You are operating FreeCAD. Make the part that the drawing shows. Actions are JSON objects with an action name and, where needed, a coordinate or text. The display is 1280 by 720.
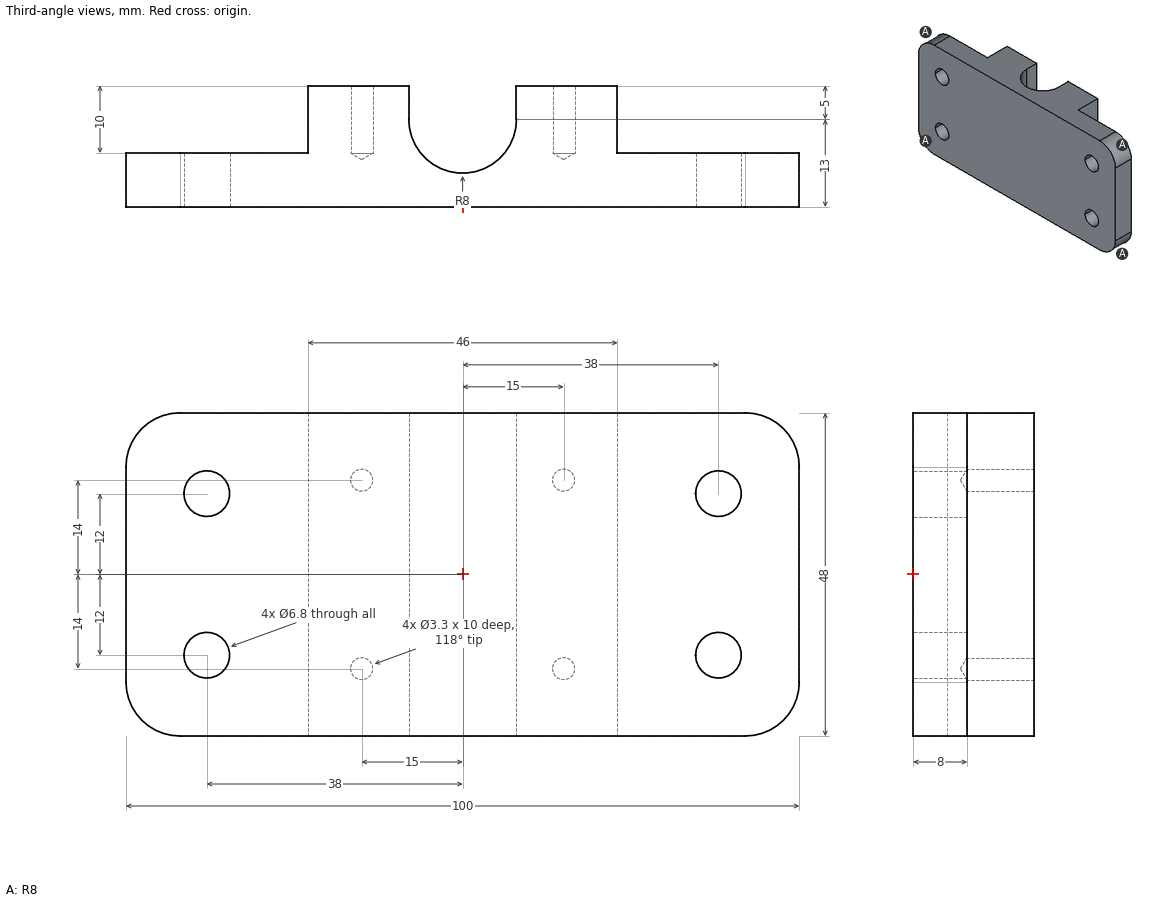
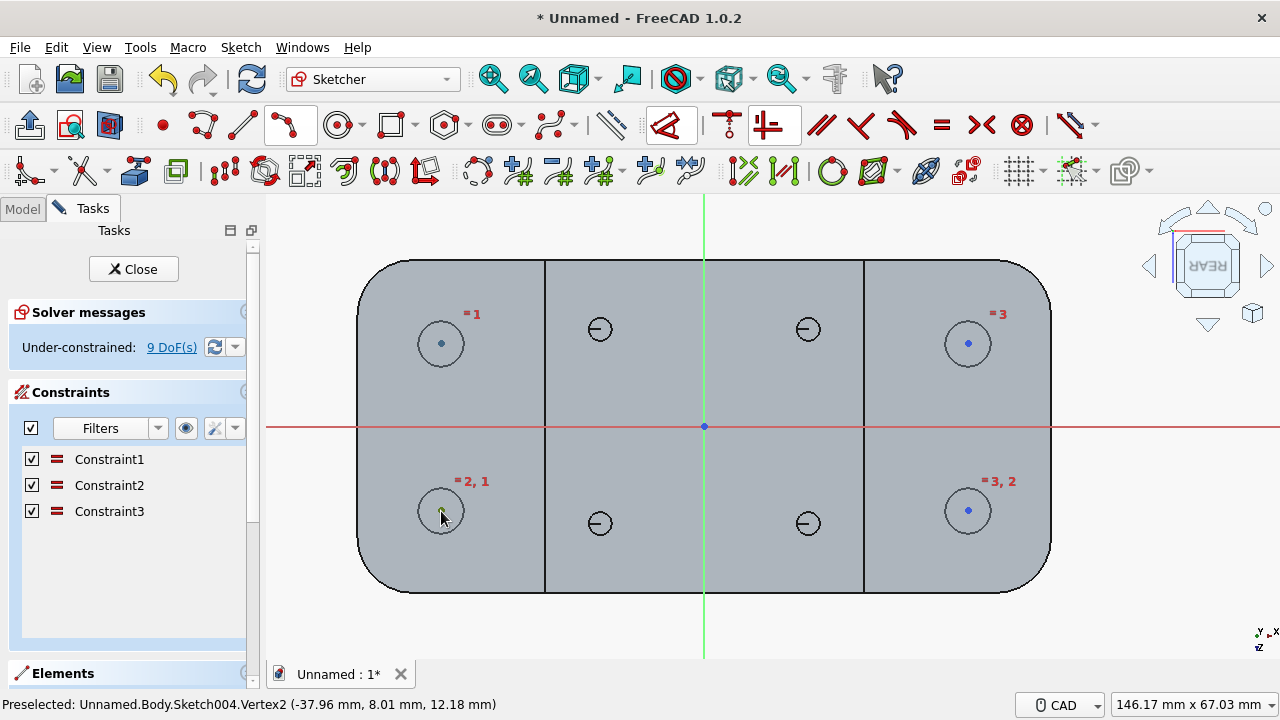
{"action": "left_click", "coordinate": [796, 126]}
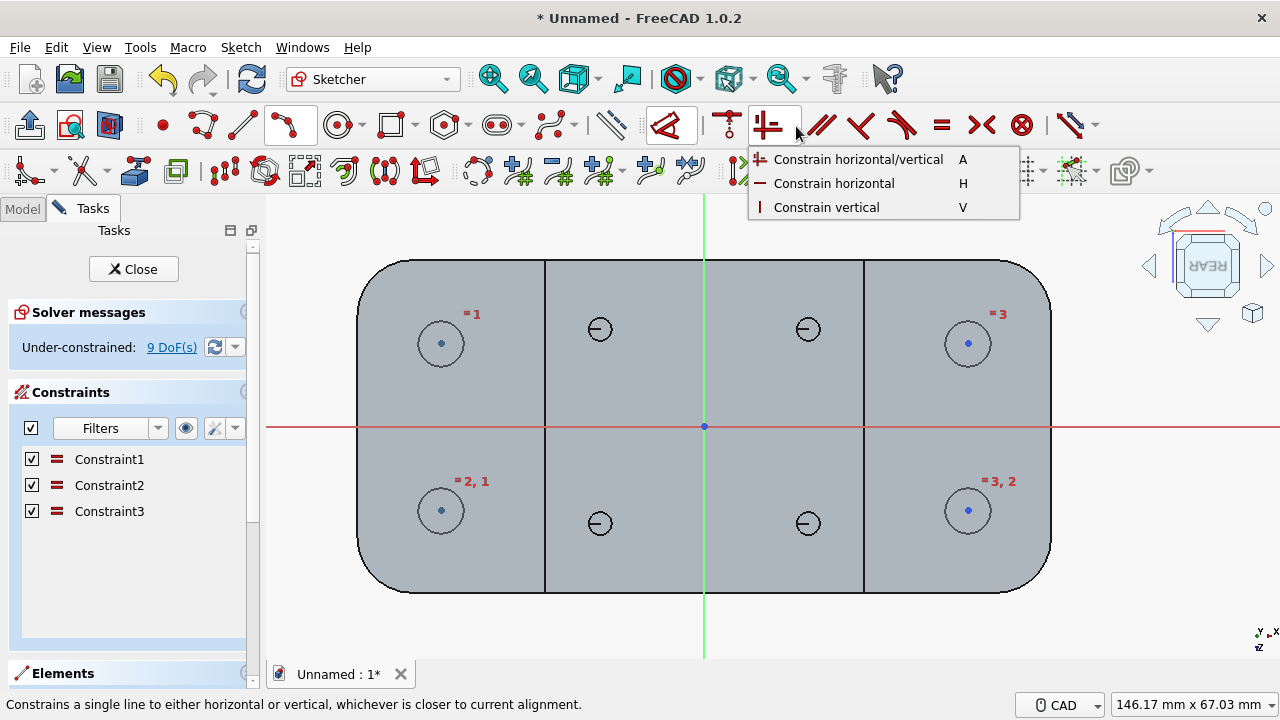
{"action": "left_click", "coordinate": [884, 207]}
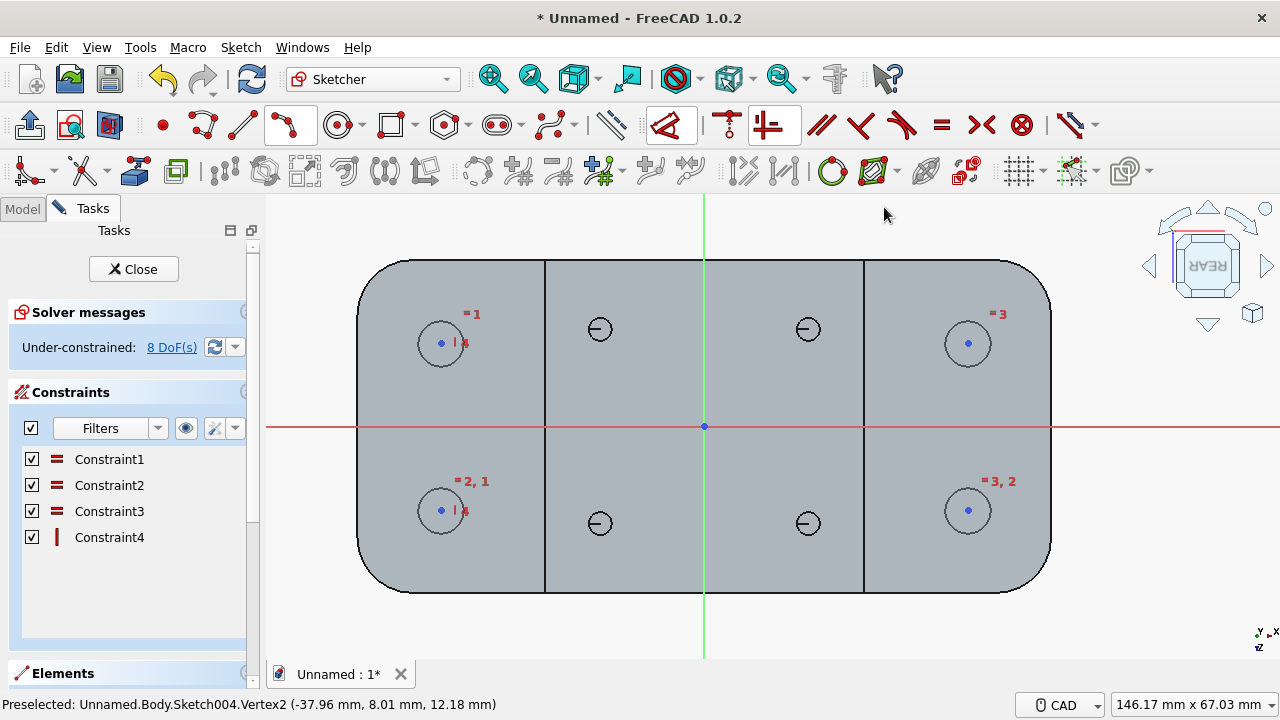
{"action": "left_click", "coordinate": [441, 511]}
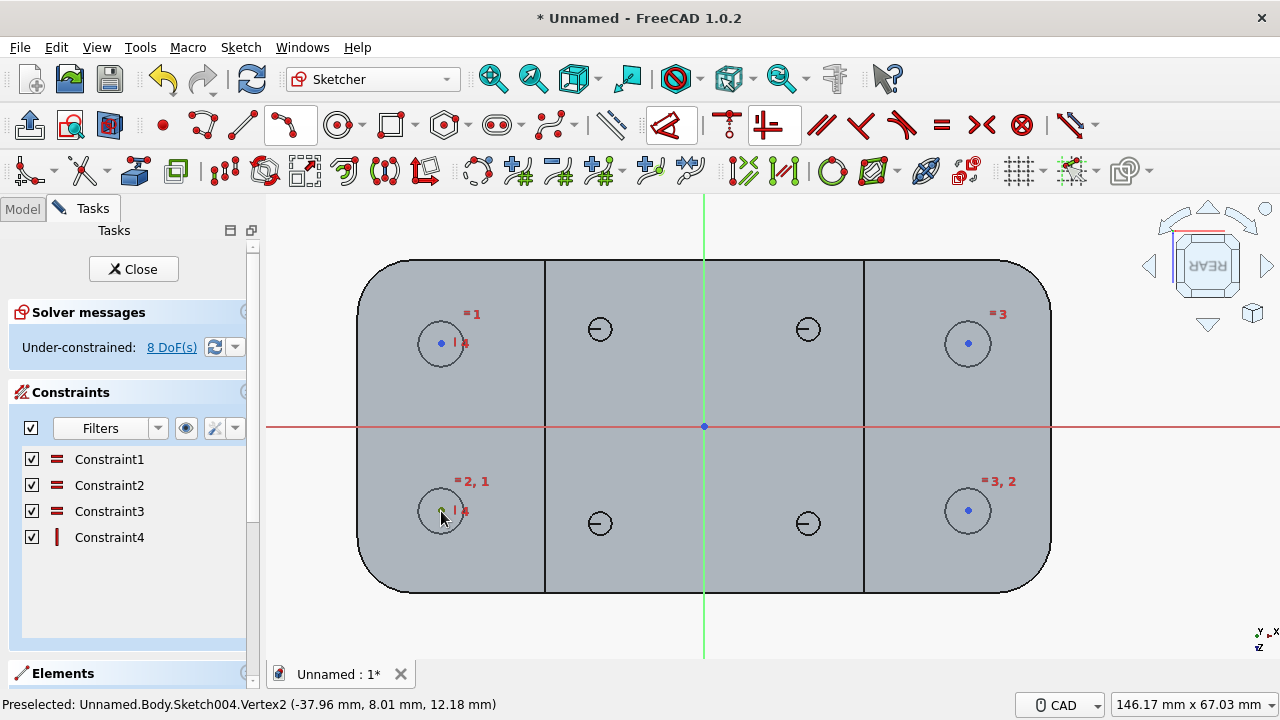
{"action": "left_click", "coordinate": [968, 511]}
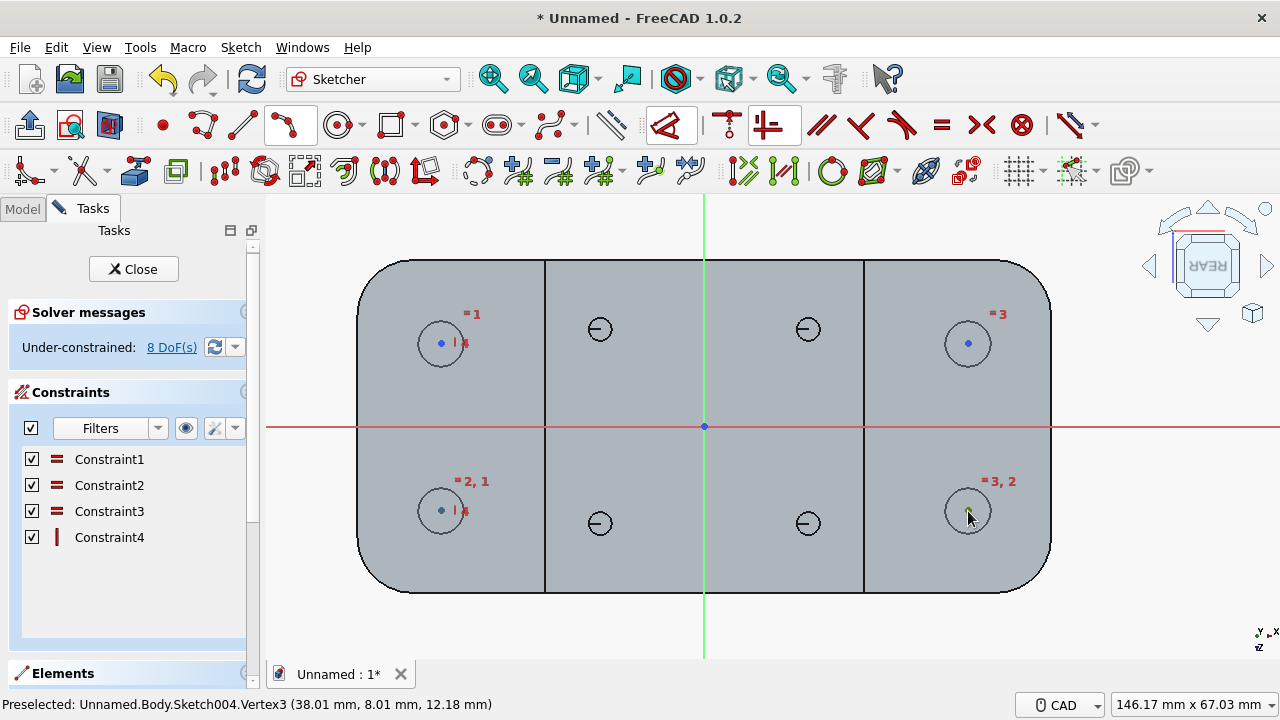
{"action": "left_click", "coordinate": [796, 126]}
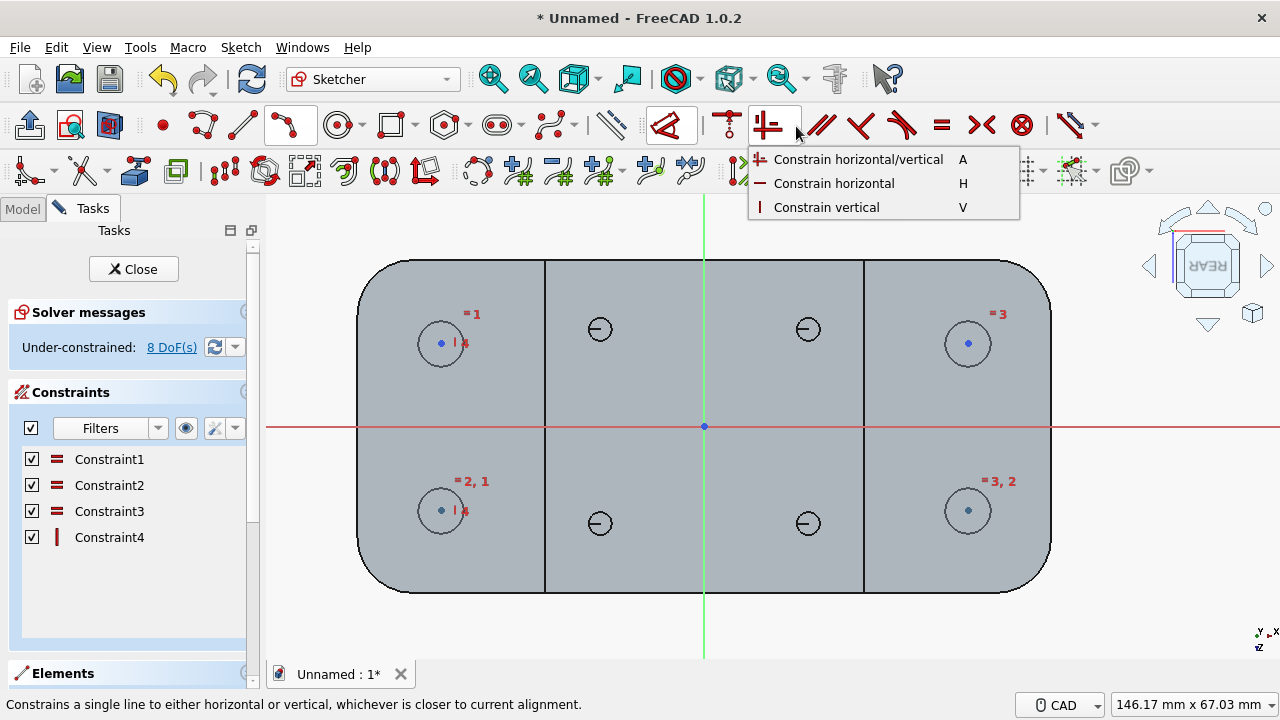
{"action": "left_click", "coordinate": [884, 183]}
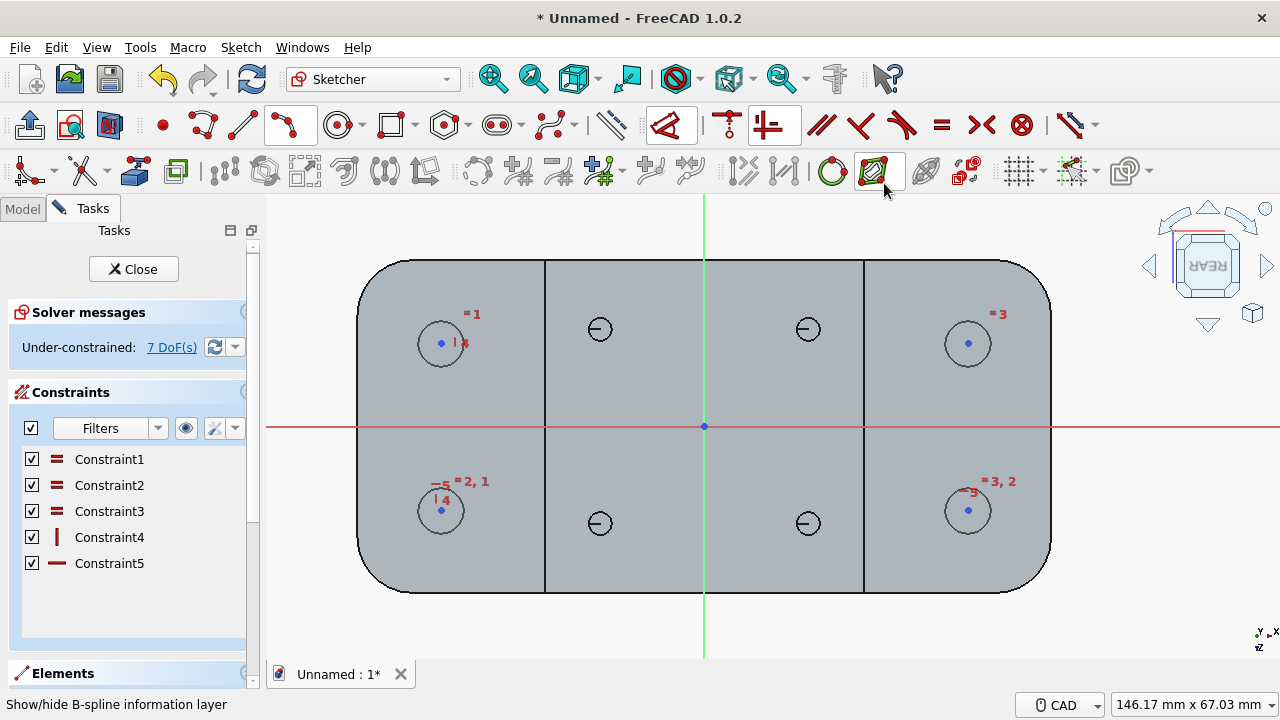
{"action": "left_click", "coordinate": [968, 511]}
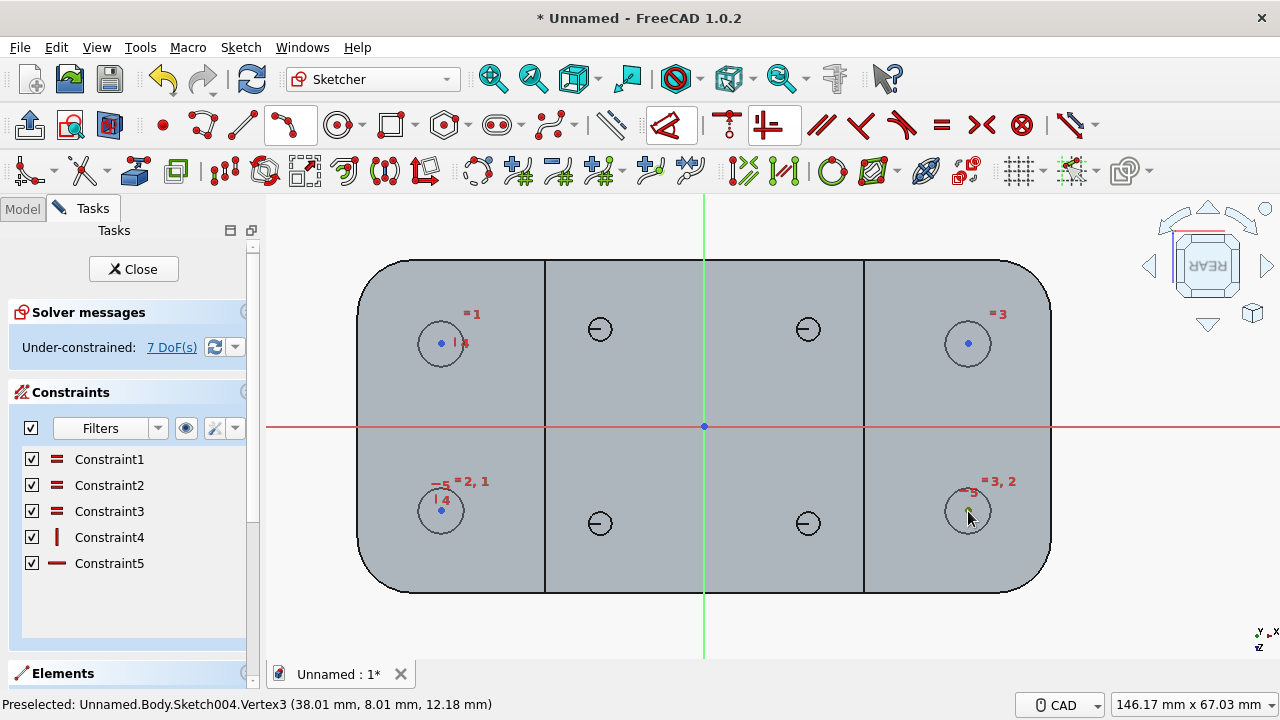
{"action": "left_click", "coordinate": [968, 344]}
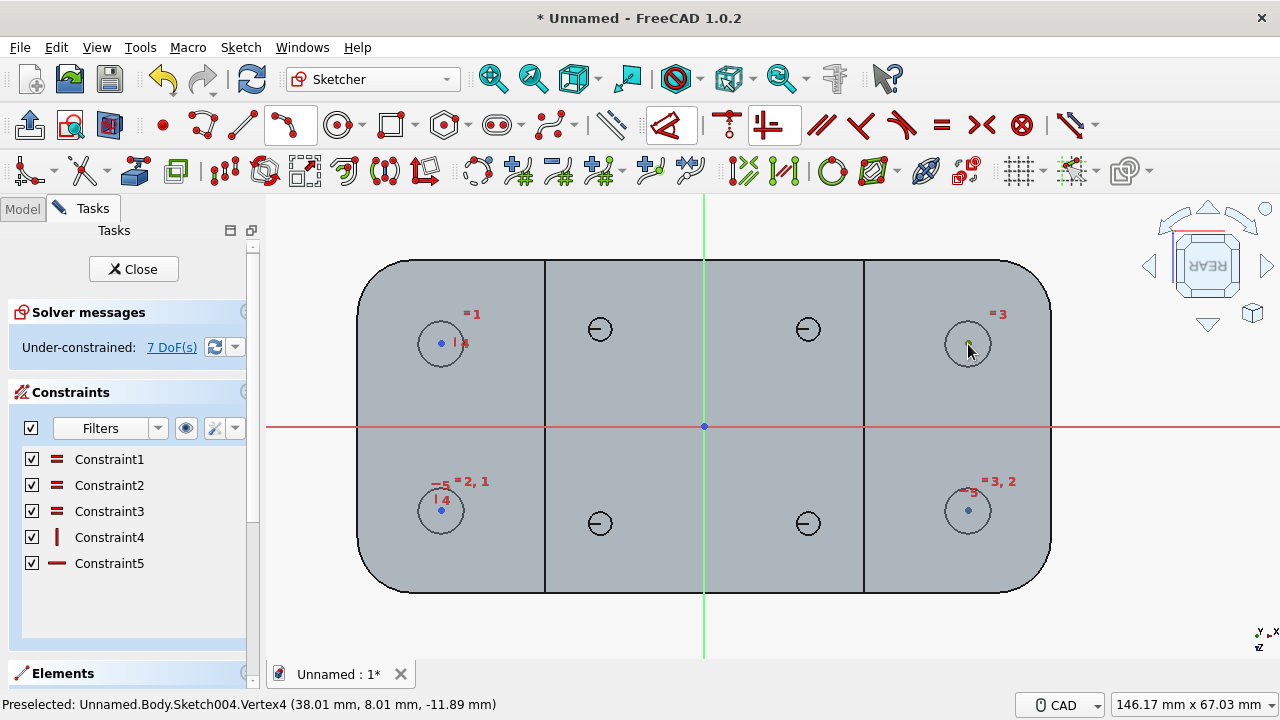
{"action": "key", "text": "v"}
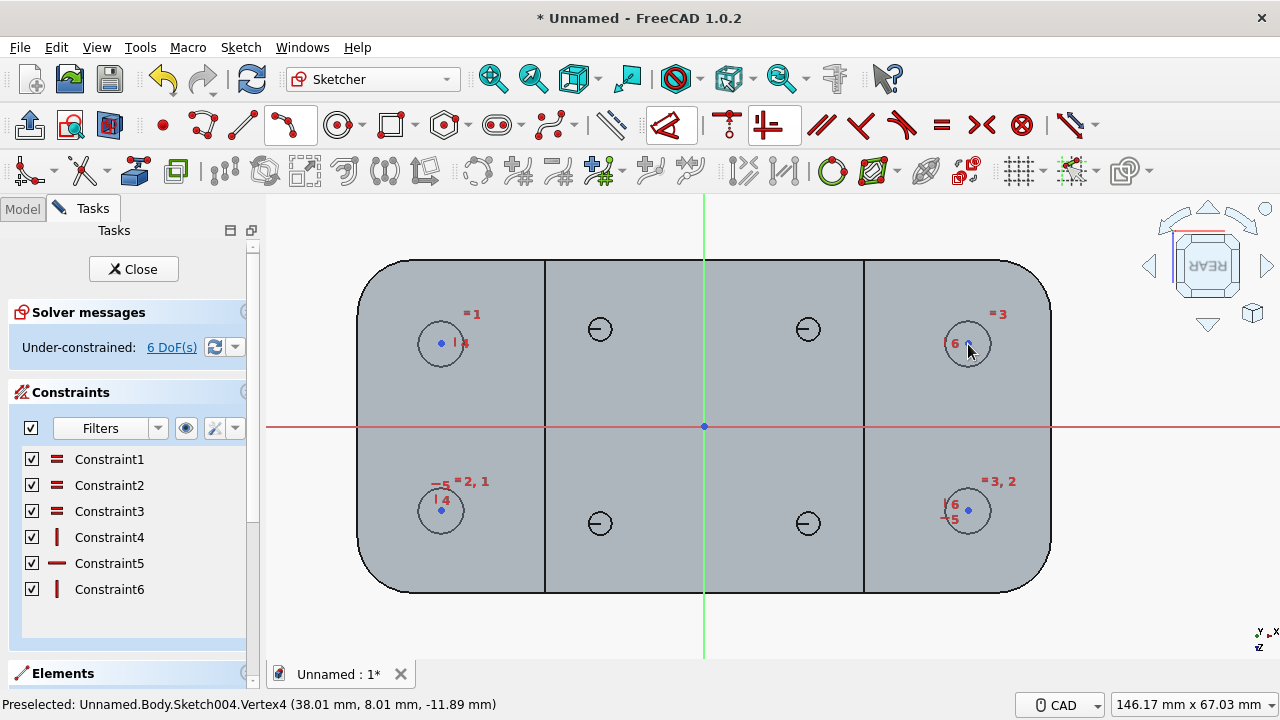
{"action": "left_click", "coordinate": [441, 344]}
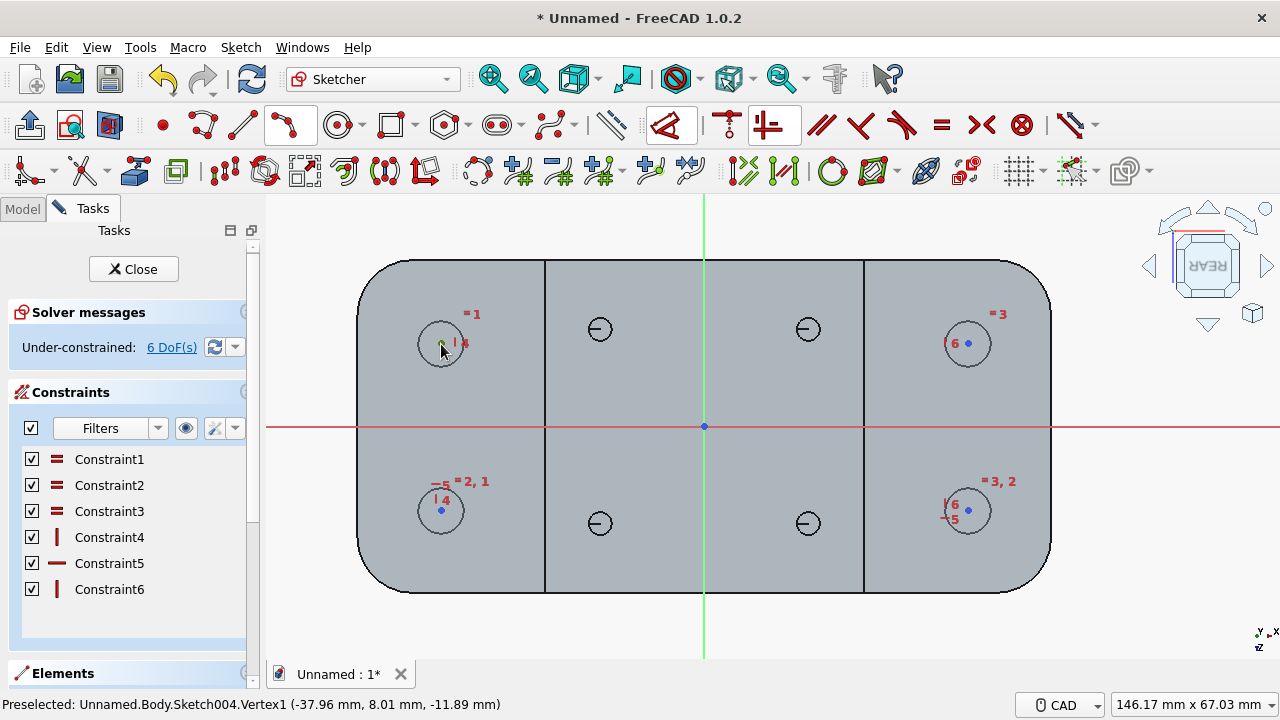
{"action": "left_click", "coordinate": [968, 344]}